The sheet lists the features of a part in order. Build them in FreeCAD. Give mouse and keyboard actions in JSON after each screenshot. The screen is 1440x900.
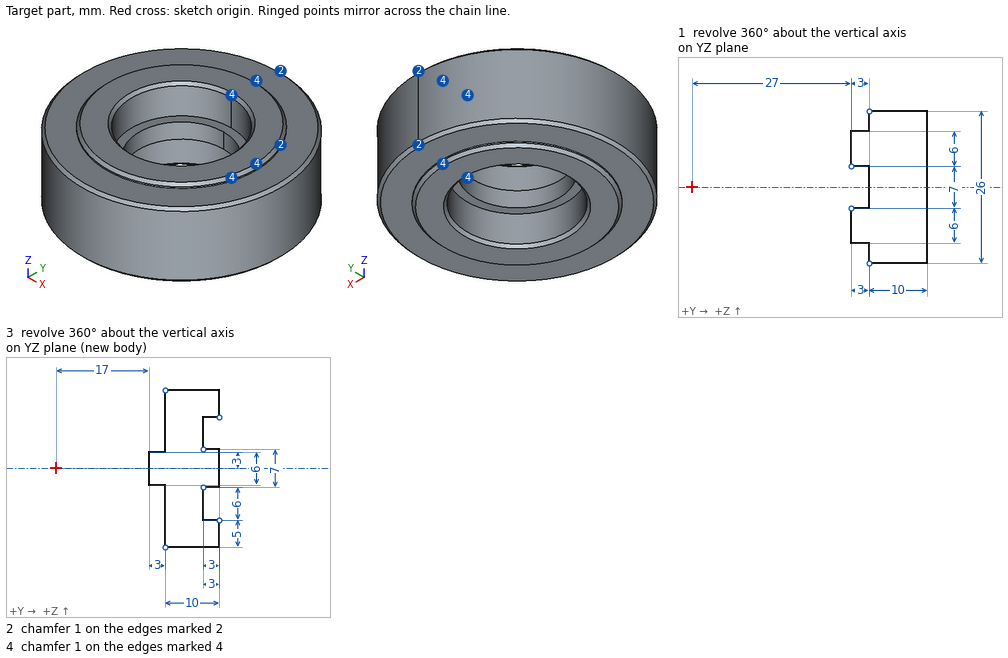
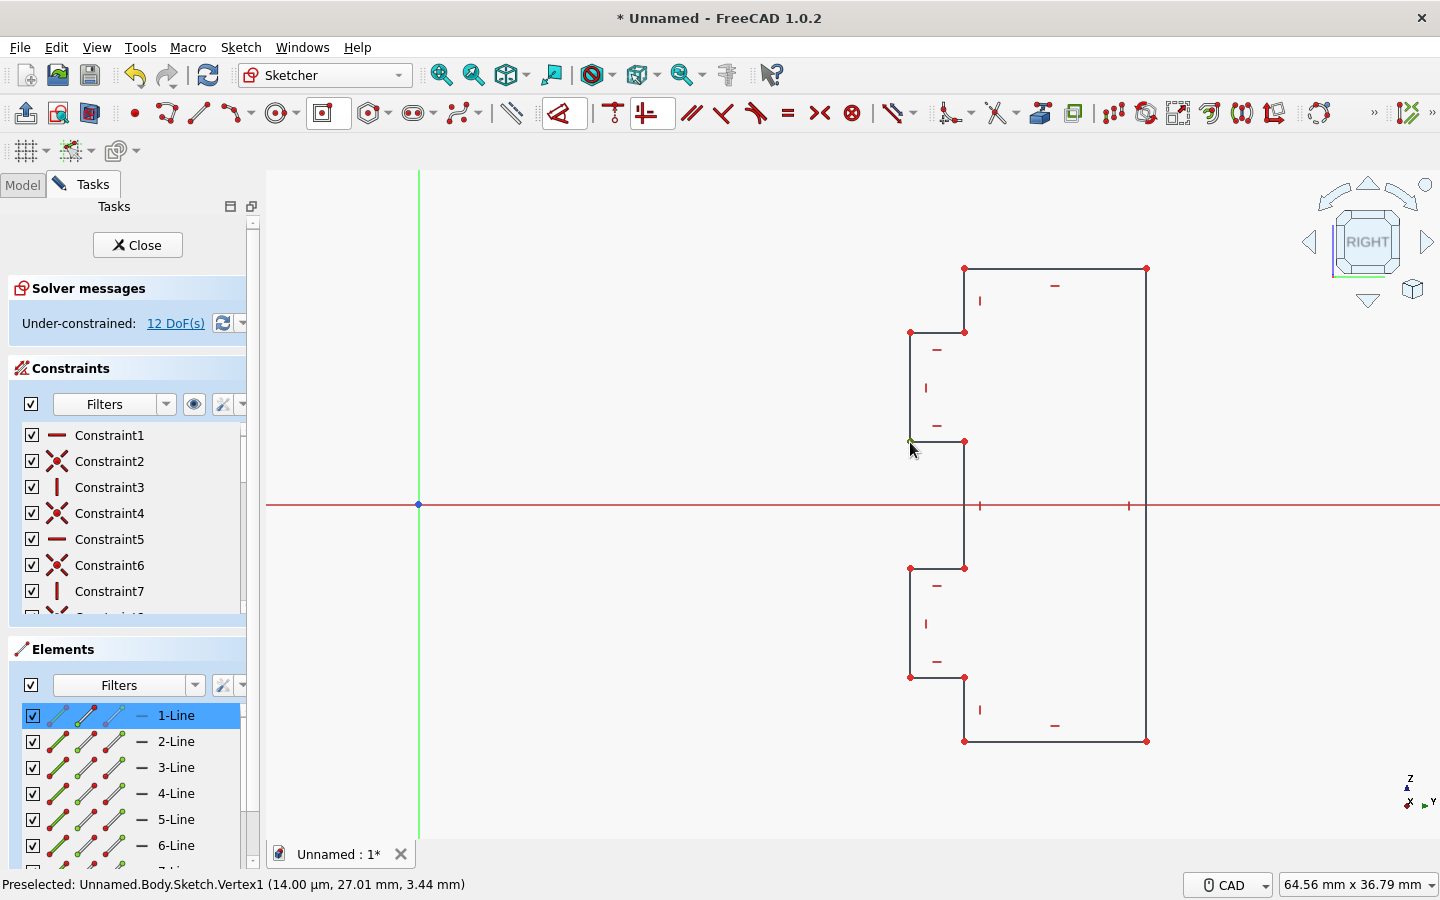
{"action": "left_click", "coordinate": [910, 569]}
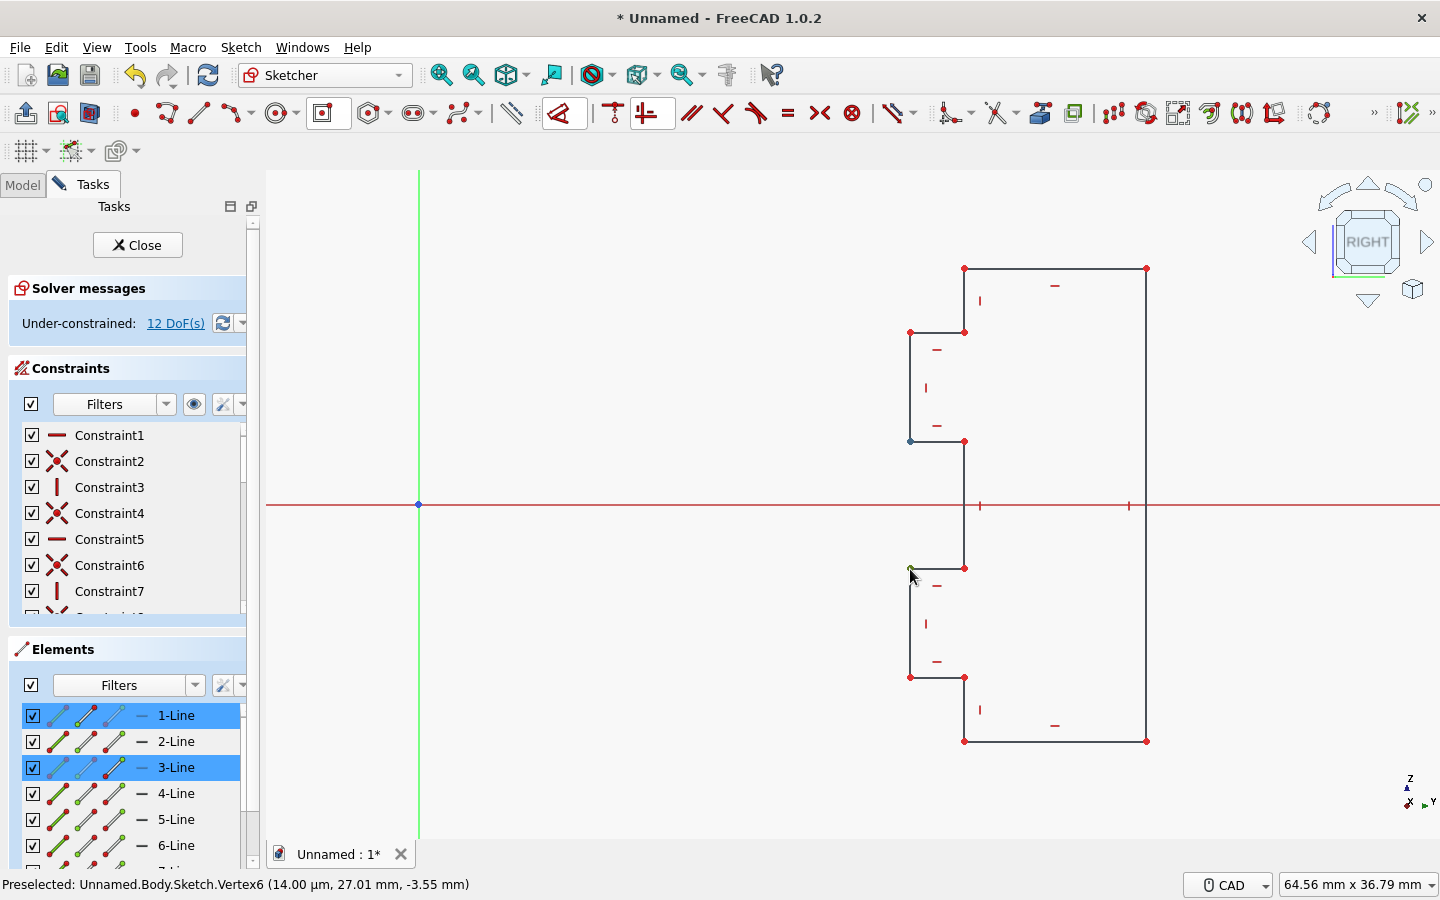
{"action": "left_click", "coordinate": [364, 504]}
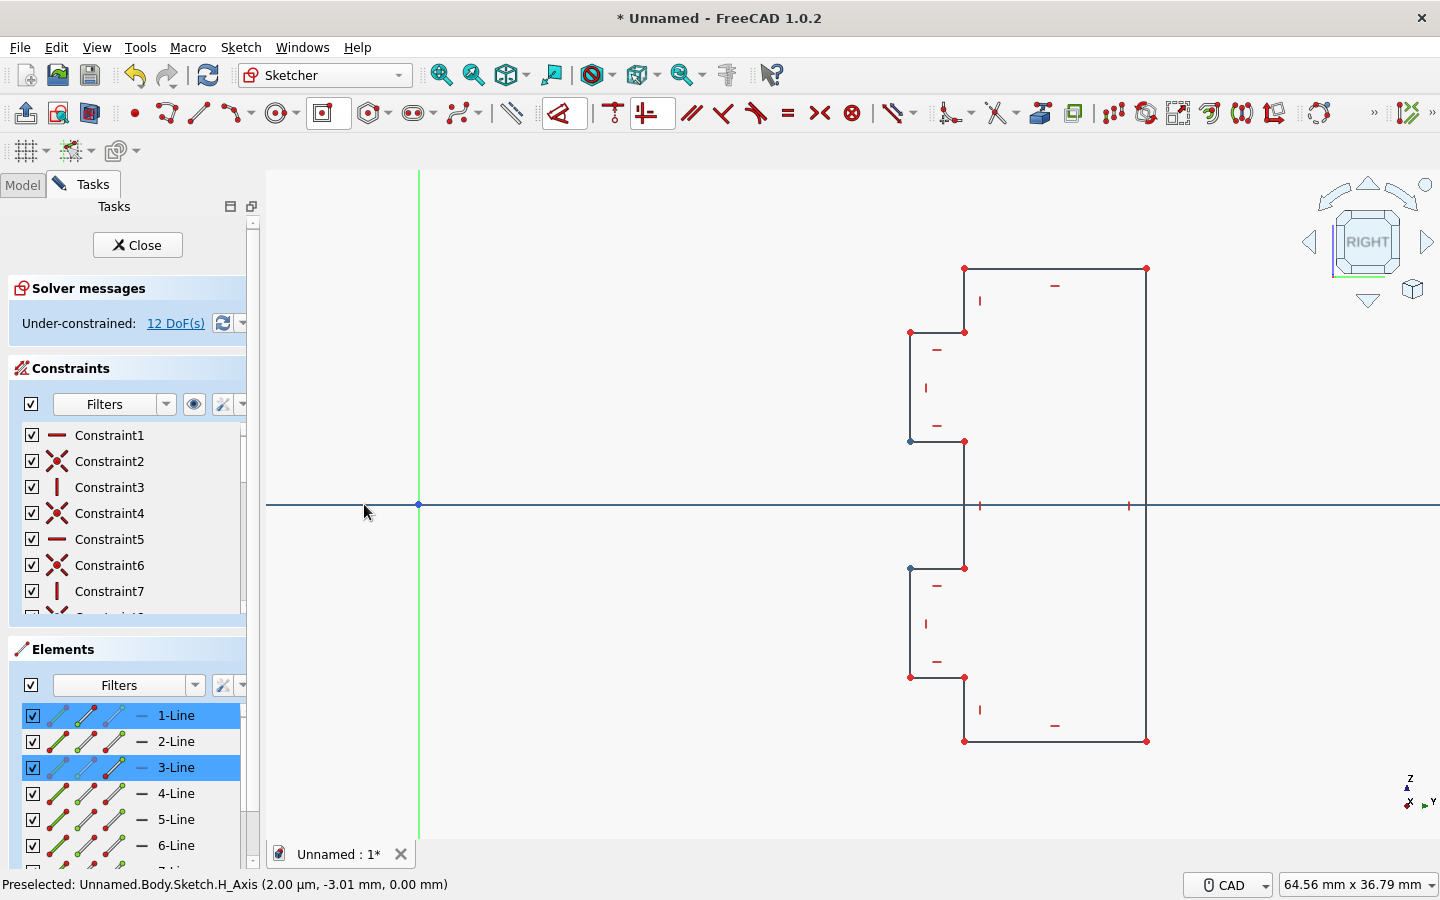
{"action": "left_click", "coordinate": [820, 114]}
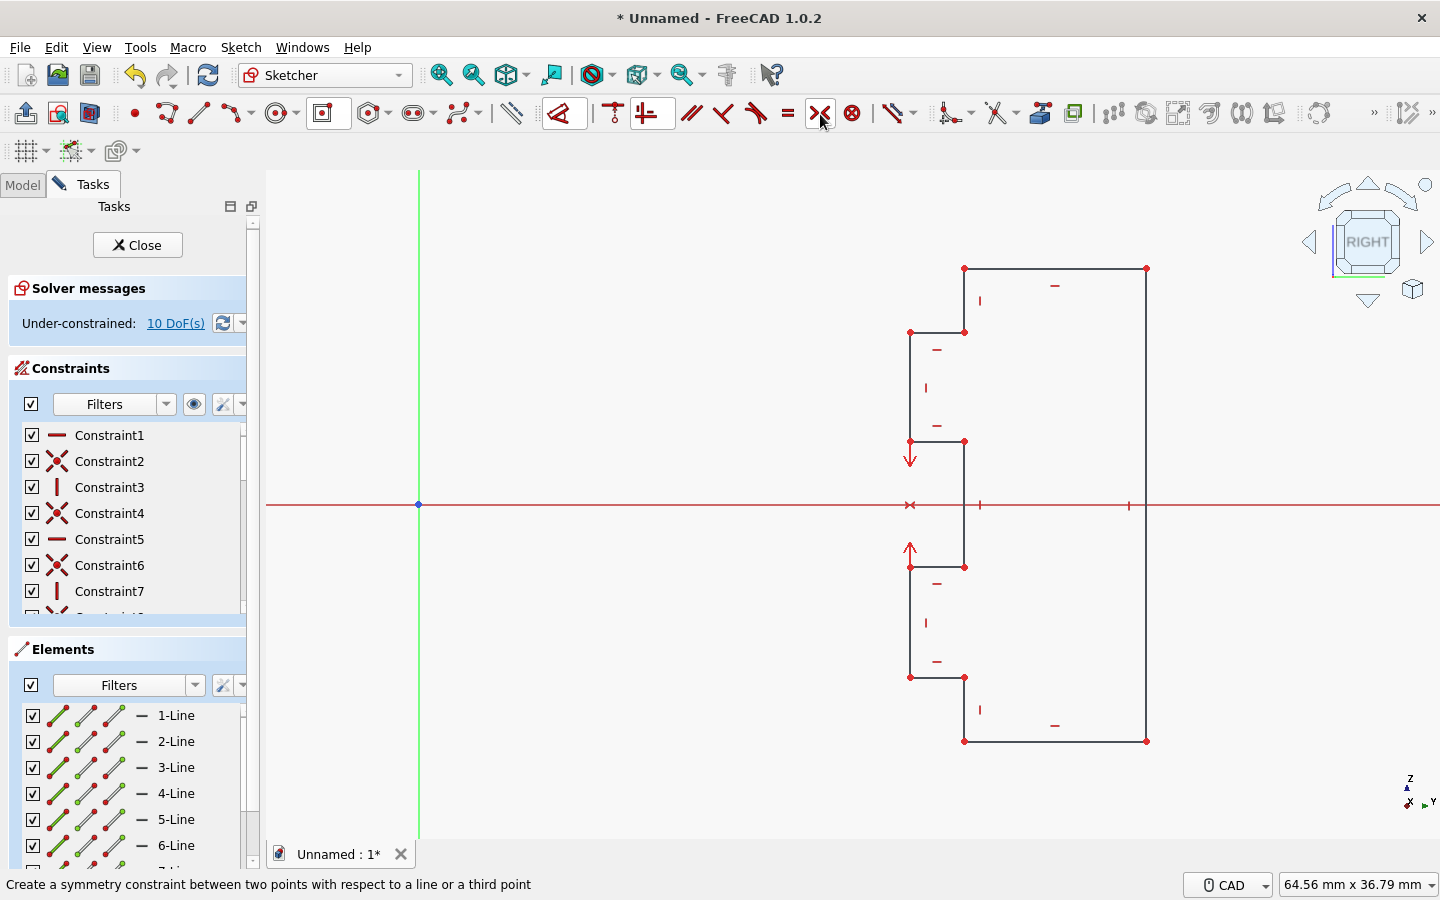
{"action": "left_click", "coordinate": [964, 742]}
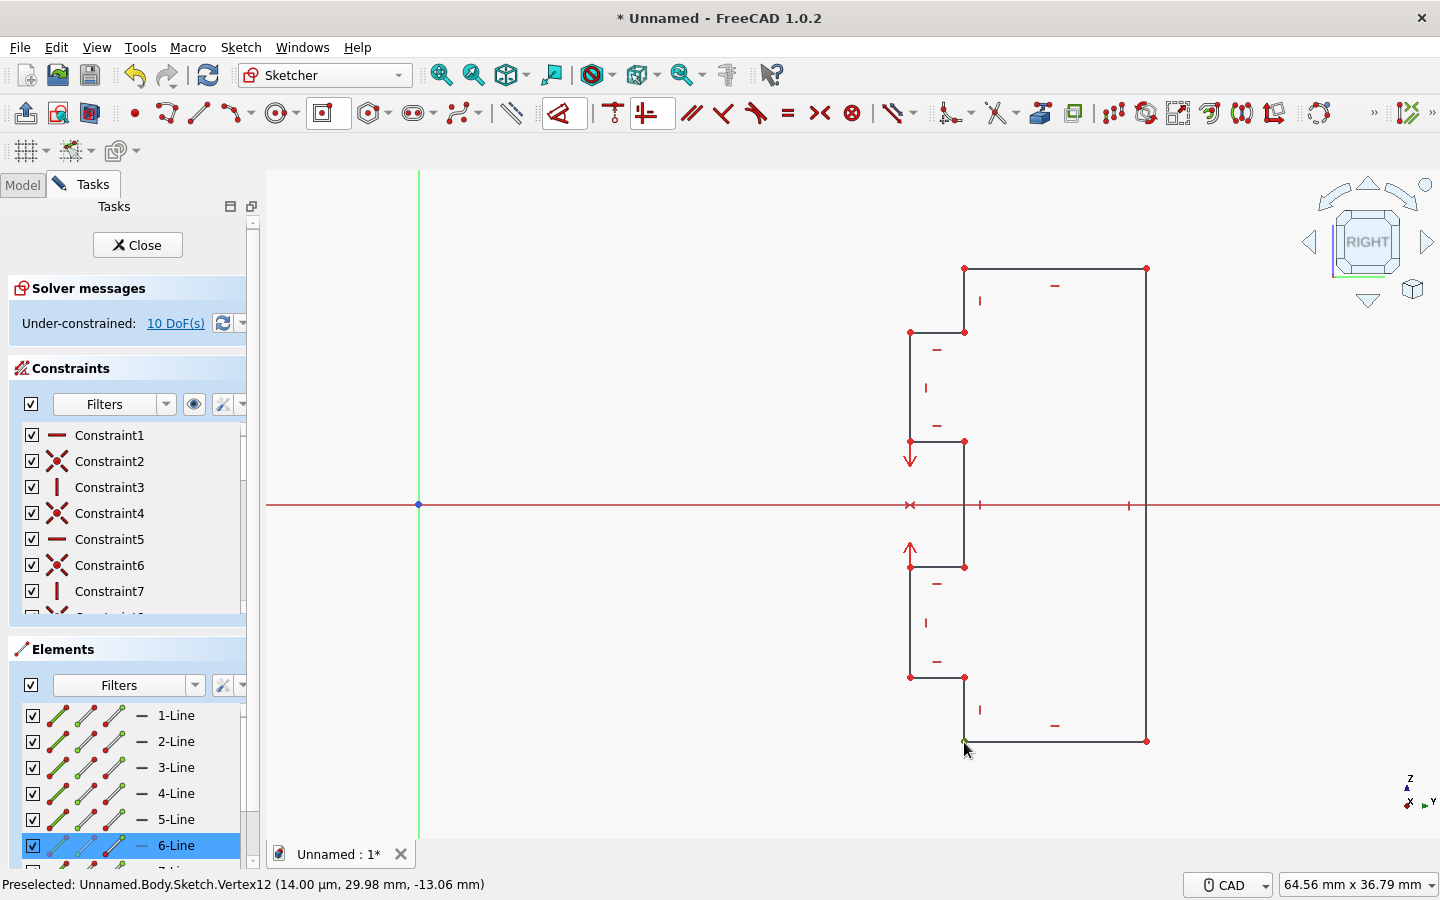
{"action": "left_click", "coordinate": [964, 269]}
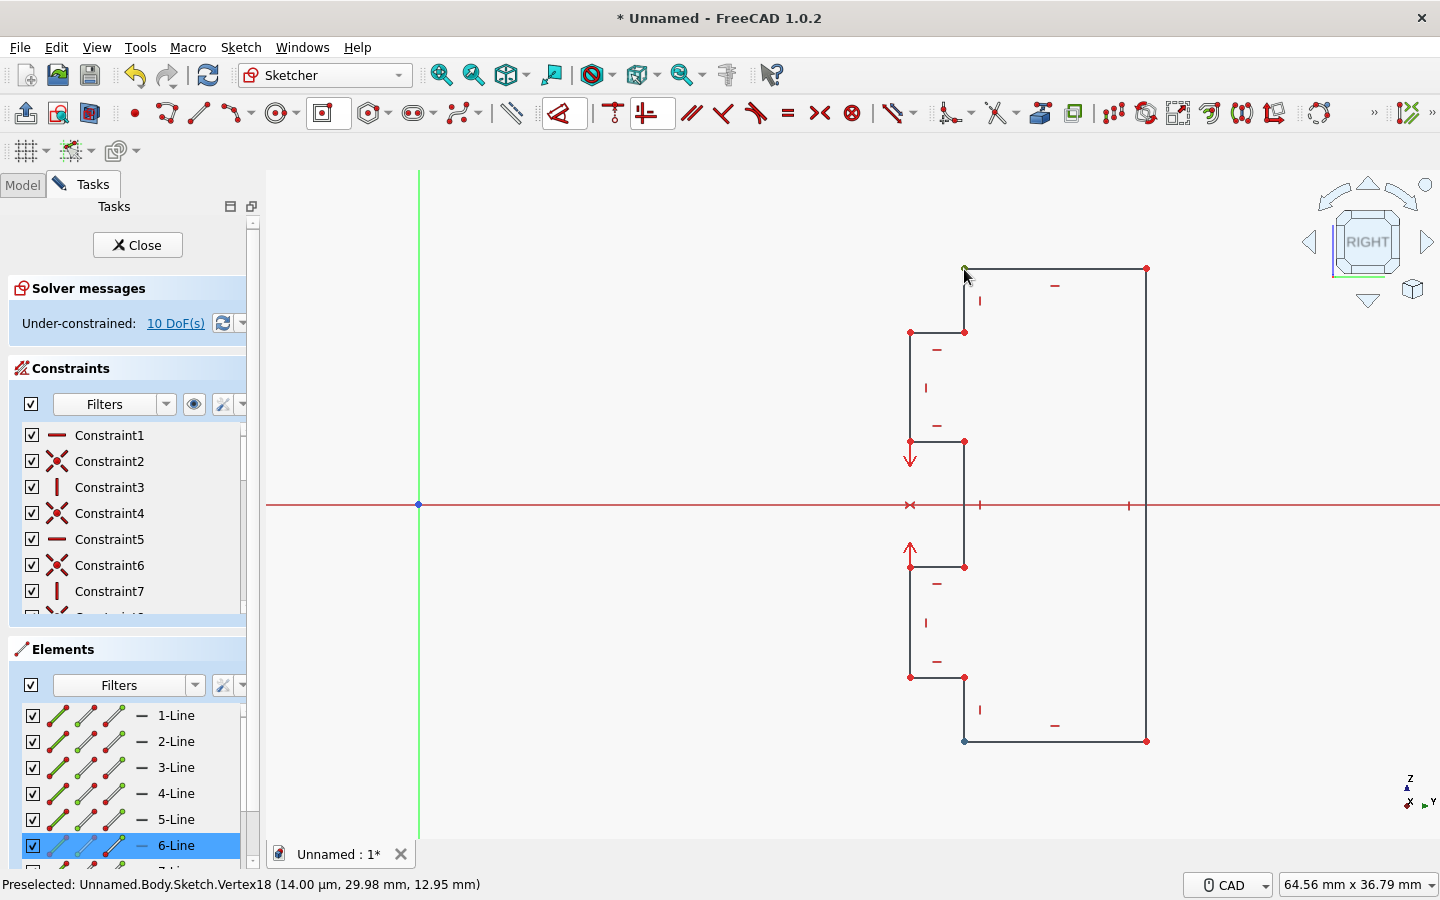
{"action": "left_click", "coordinate": [364, 504]}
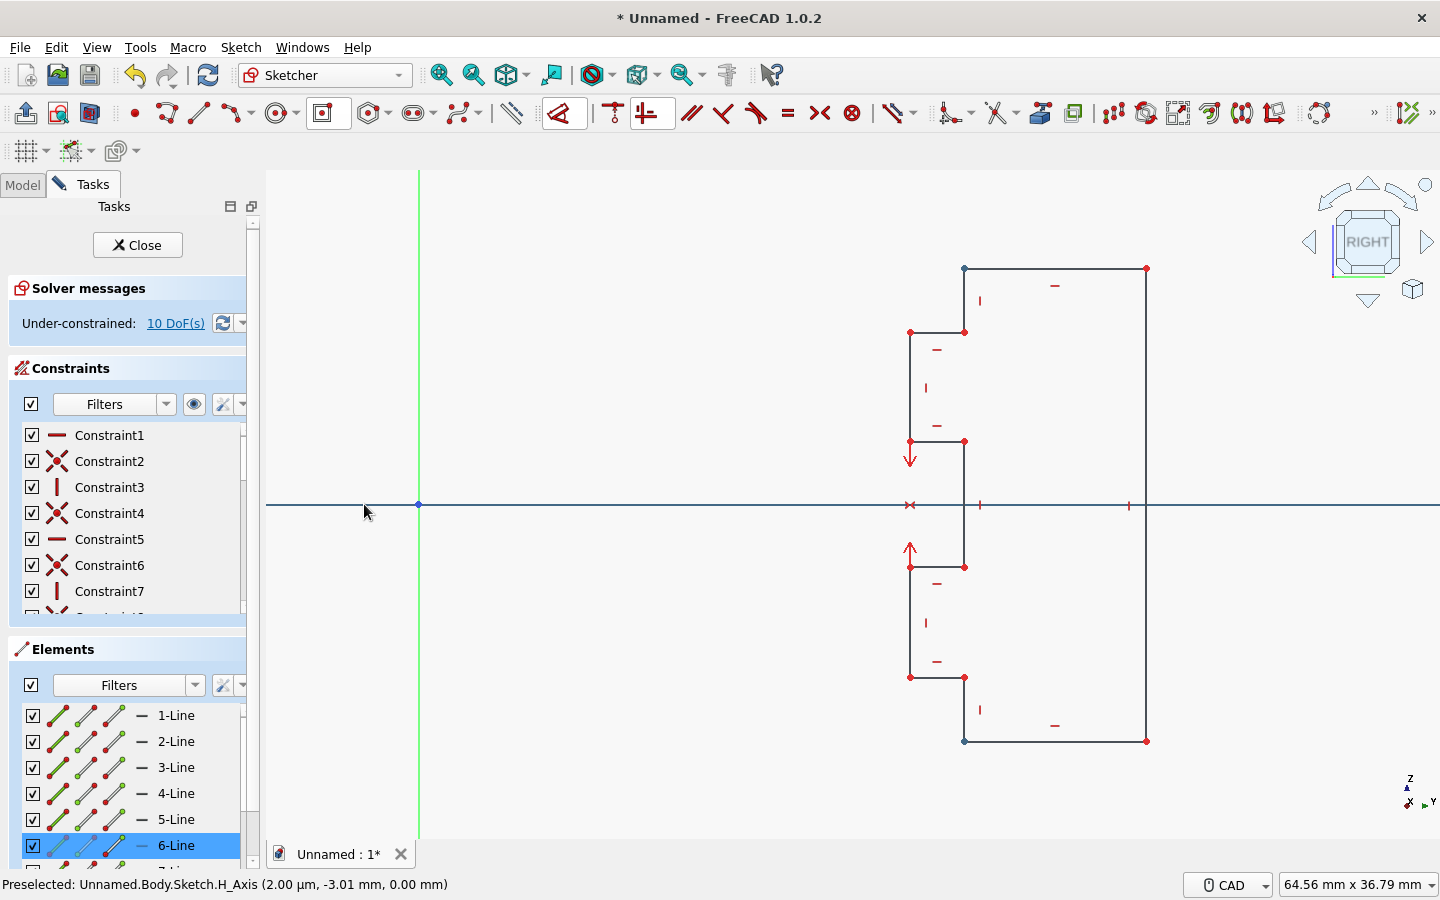
{"action": "left_click", "coordinate": [820, 114]}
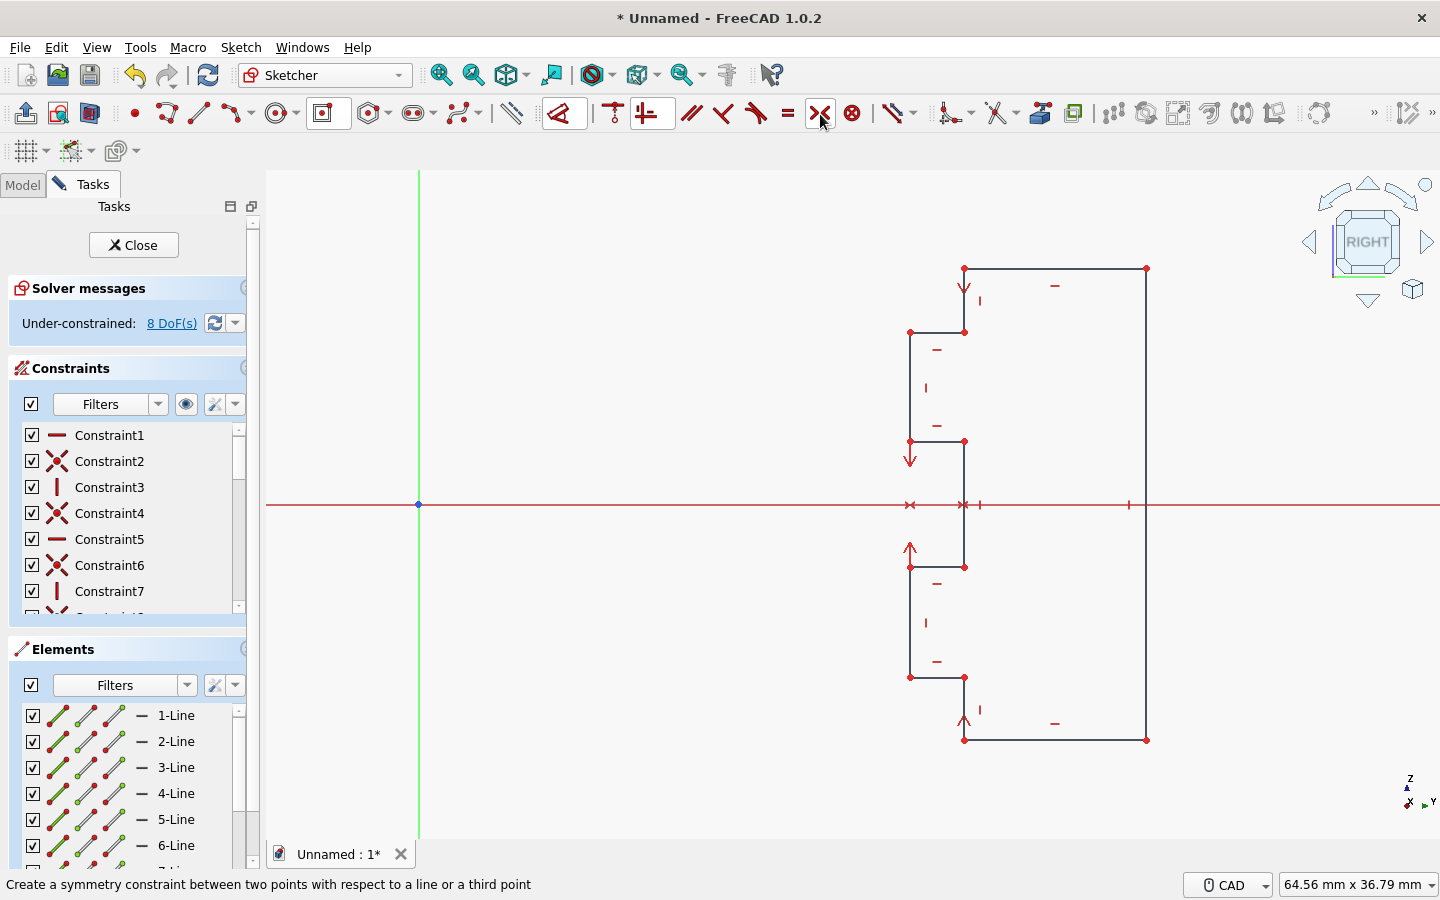
{"action": "left_click", "coordinate": [558, 114]}